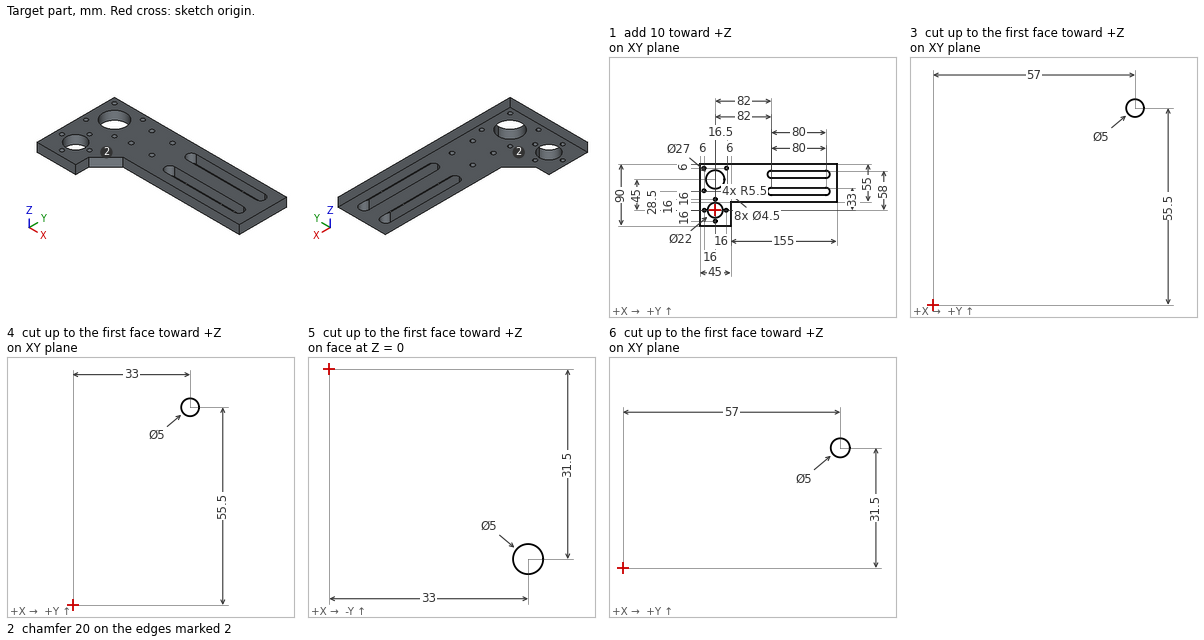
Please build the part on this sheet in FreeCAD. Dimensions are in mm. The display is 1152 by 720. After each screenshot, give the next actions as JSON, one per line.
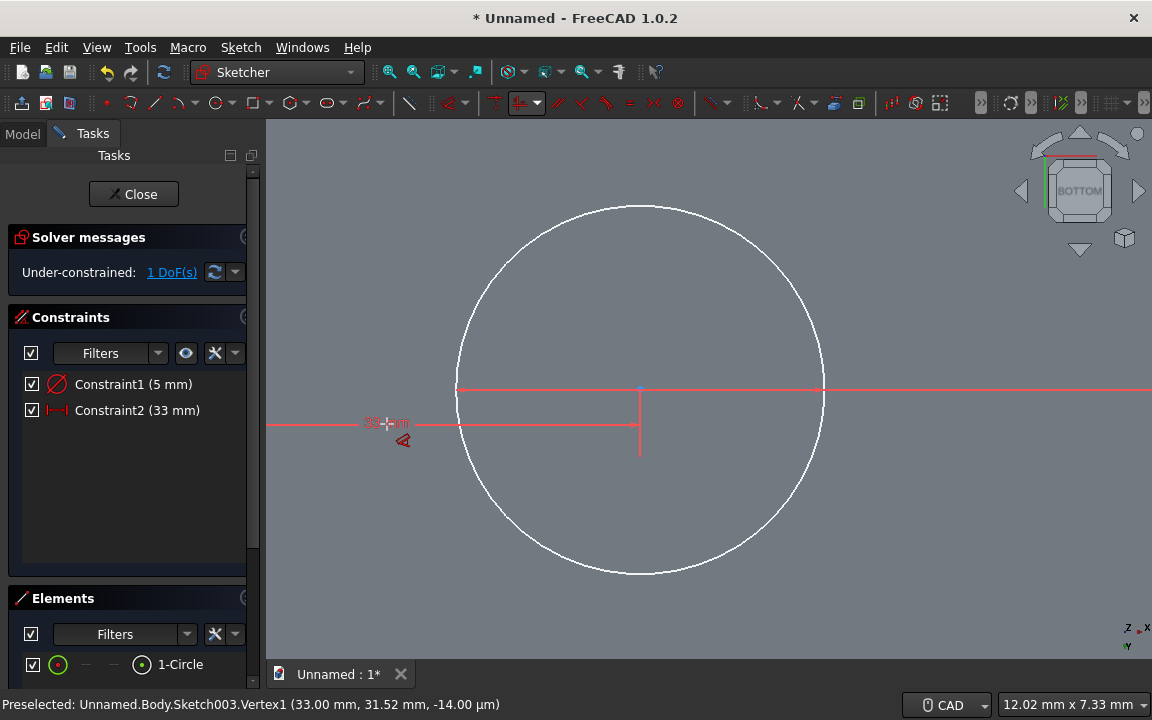
{"action": "left_click", "coordinate": [640, 390]}
{"action": "left_click", "coordinate": [674, 269]}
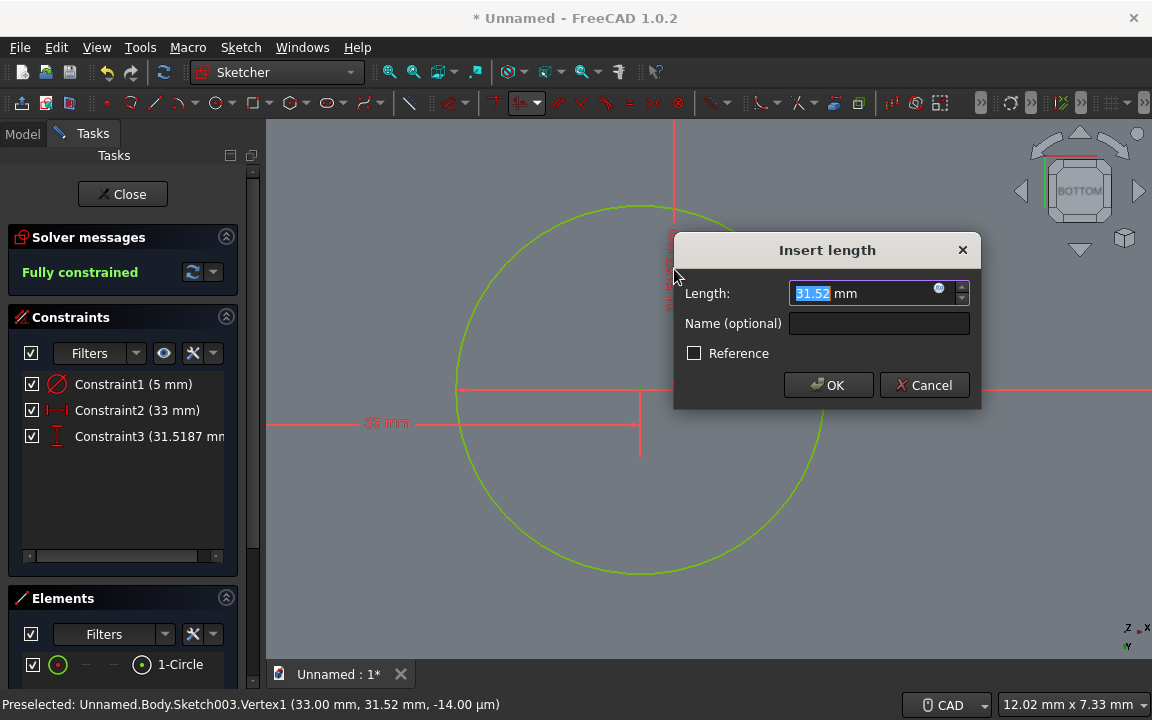
{"action": "type", "text": "31.5"}
{"action": "key", "text": "Return"}
{"action": "key", "text": "Escape"}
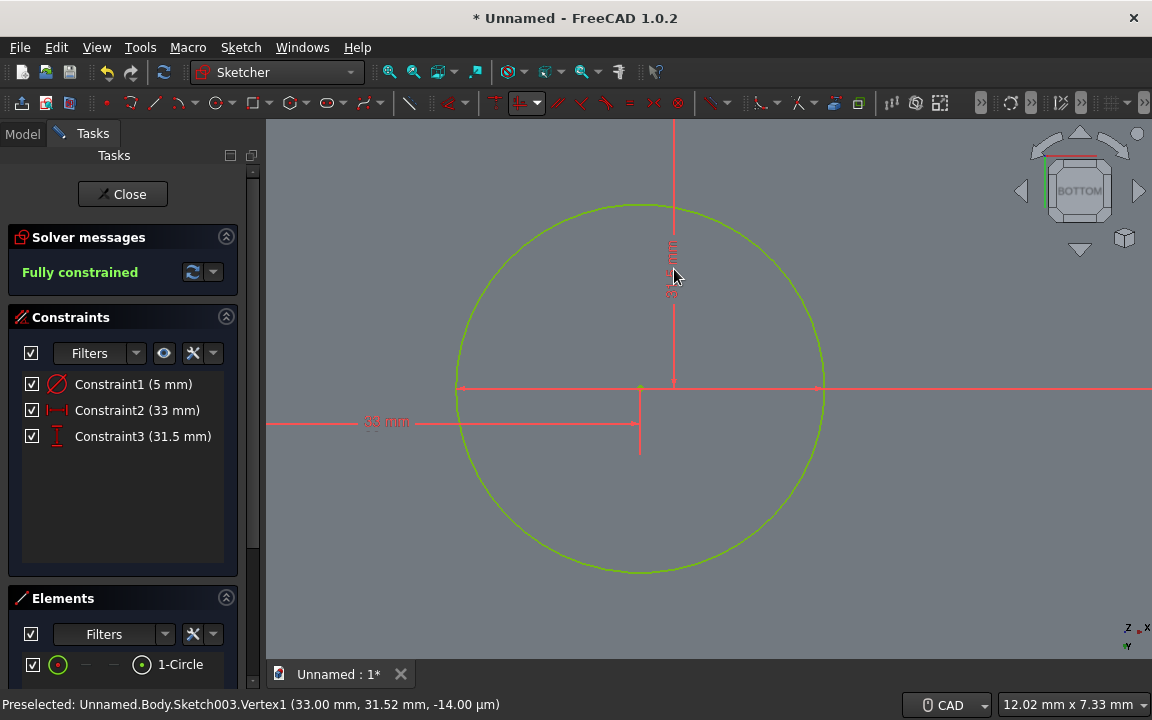
{"action": "left_click", "coordinate": [123, 194]}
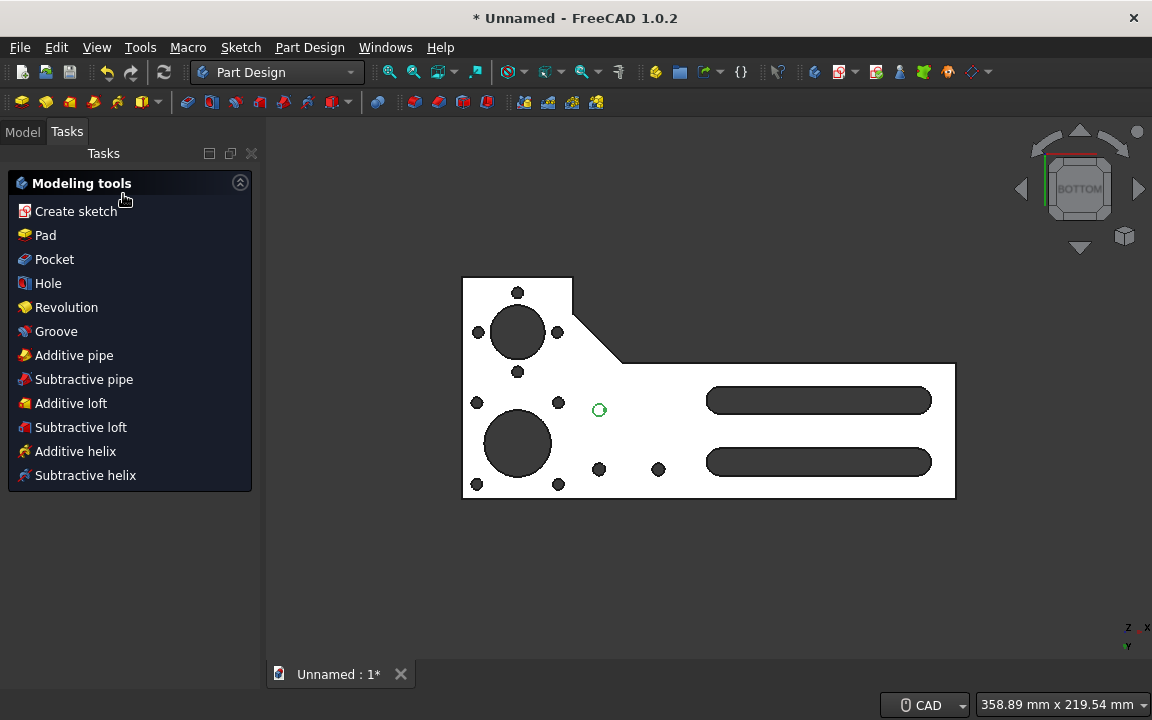
{"action": "left_click", "coordinate": [188, 102]}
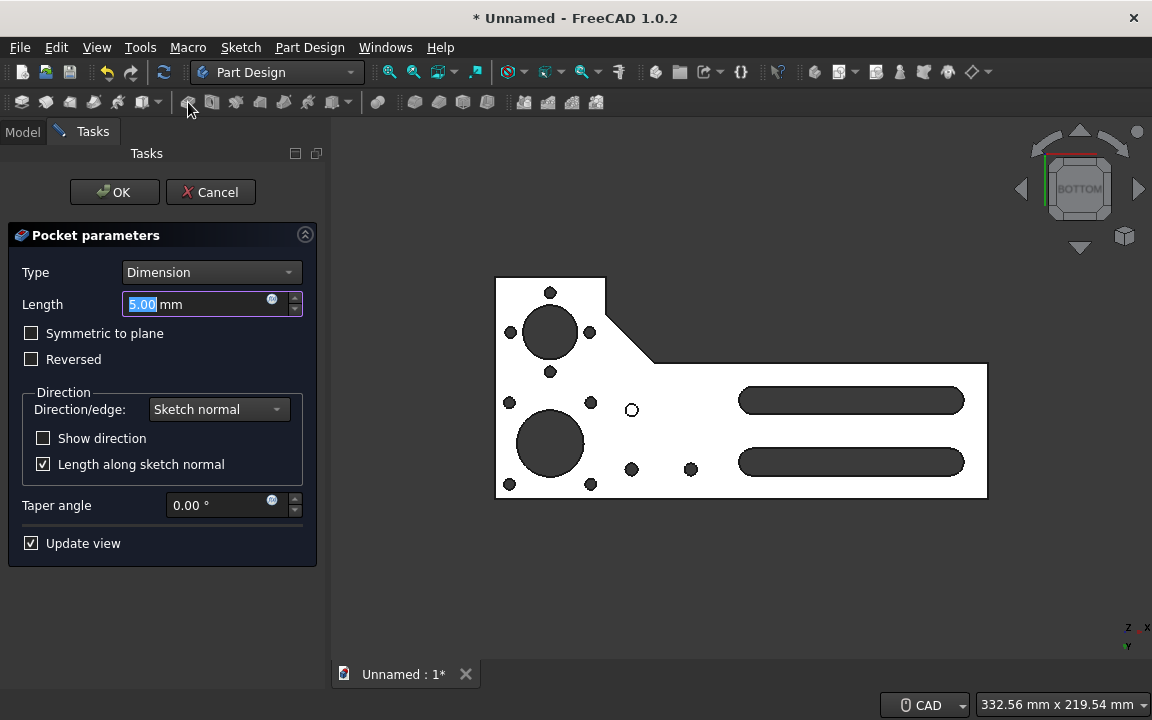
{"action": "left_click", "coordinate": [212, 272]}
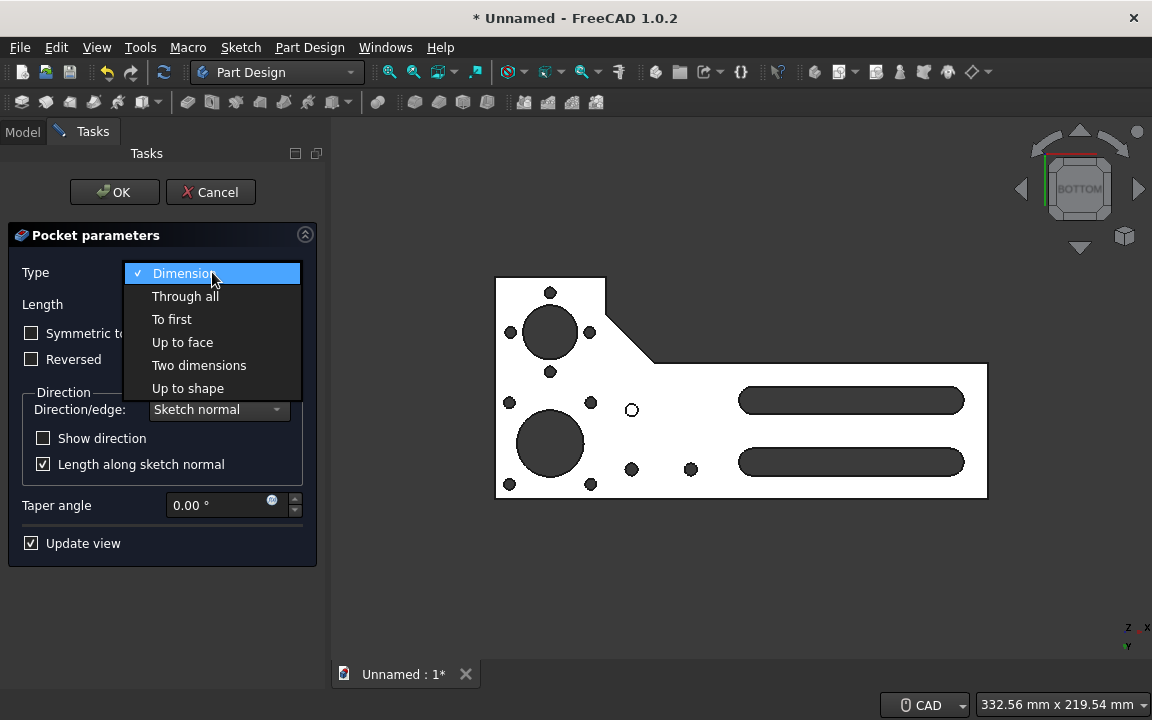
{"action": "left_click", "coordinate": [212, 320]}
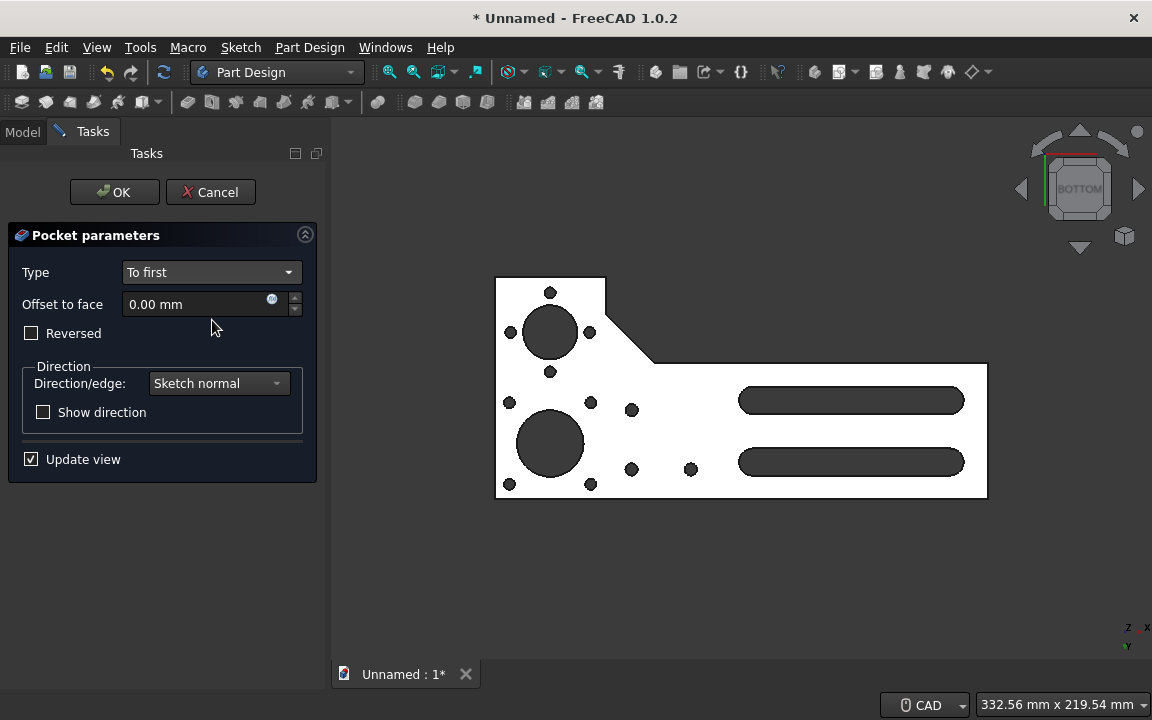
{"action": "left_click", "coordinate": [115, 192]}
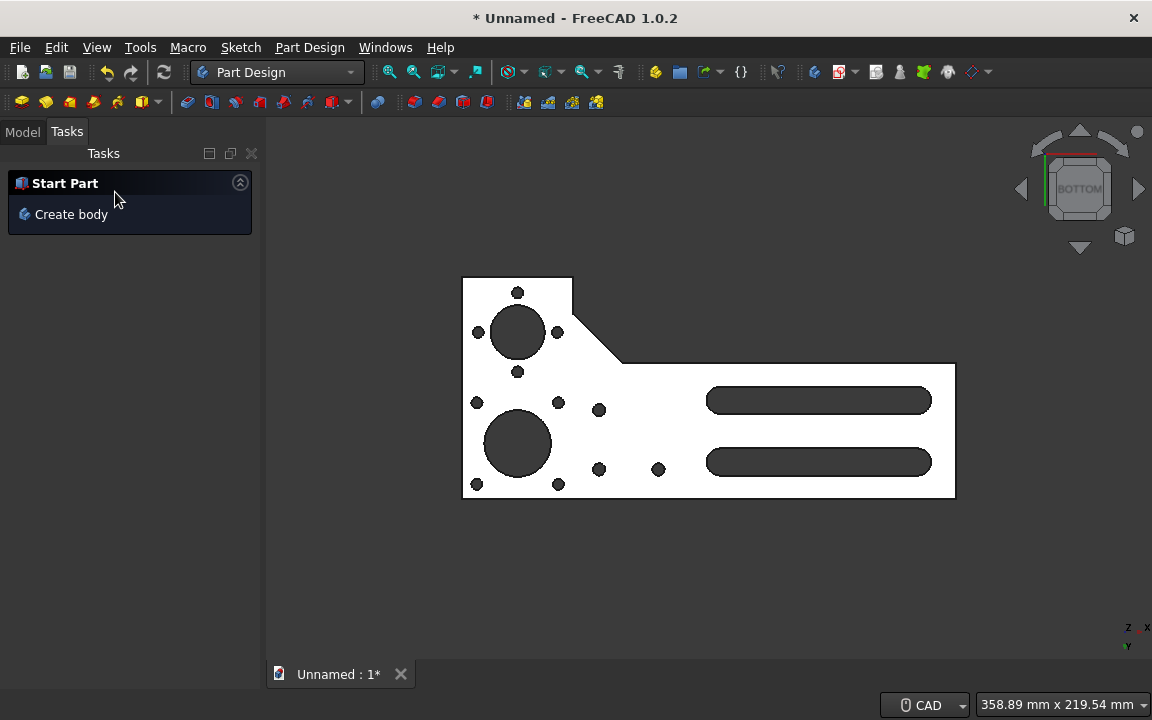
{"action": "left_click", "coordinate": [840, 72]}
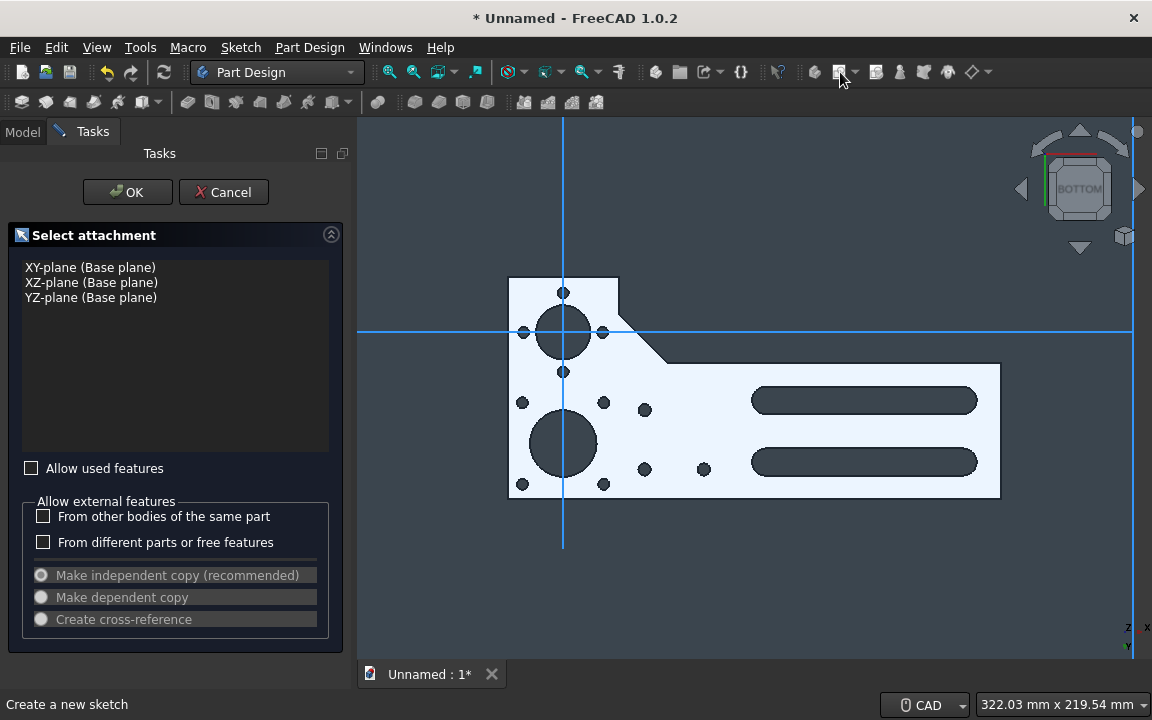
{"action": "left_click", "coordinate": [82, 268]}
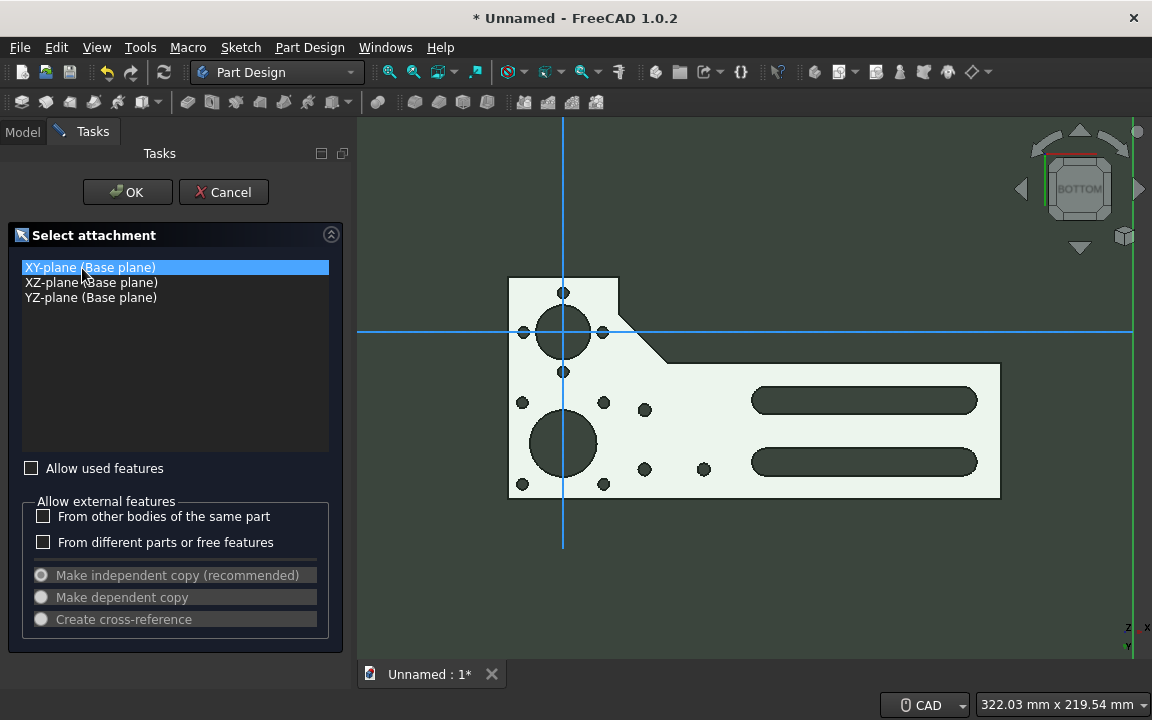
{"action": "left_click", "coordinate": [128, 192]}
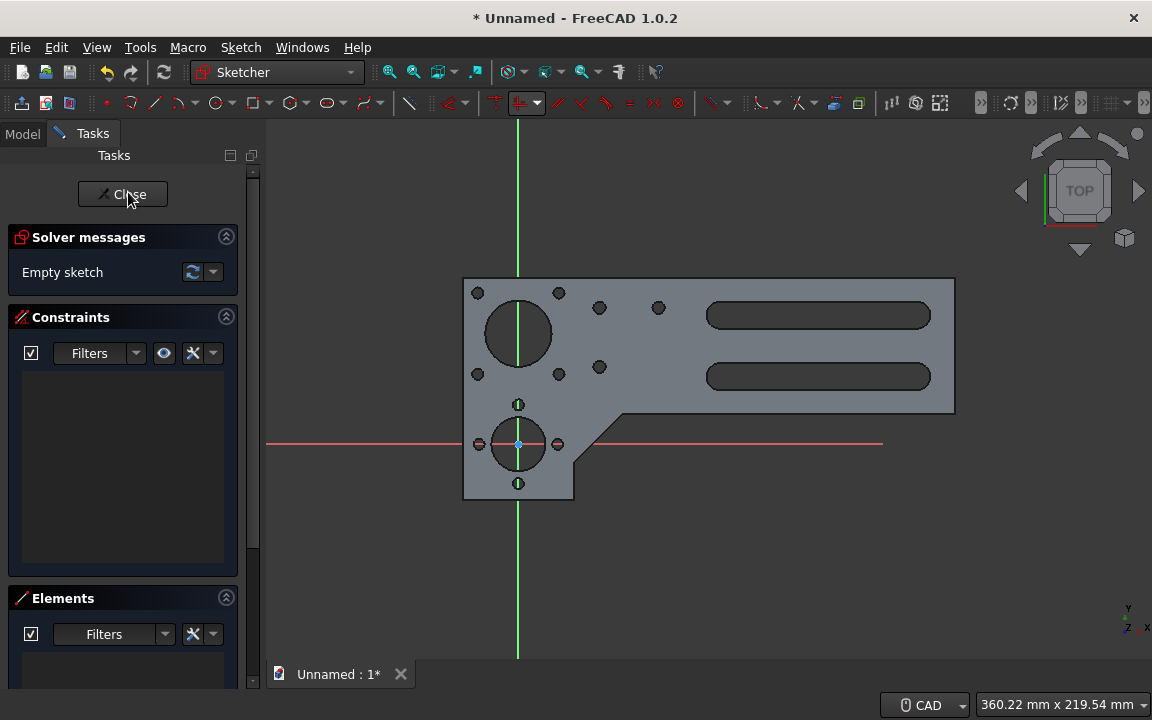
{"action": "key", "text": "q s"}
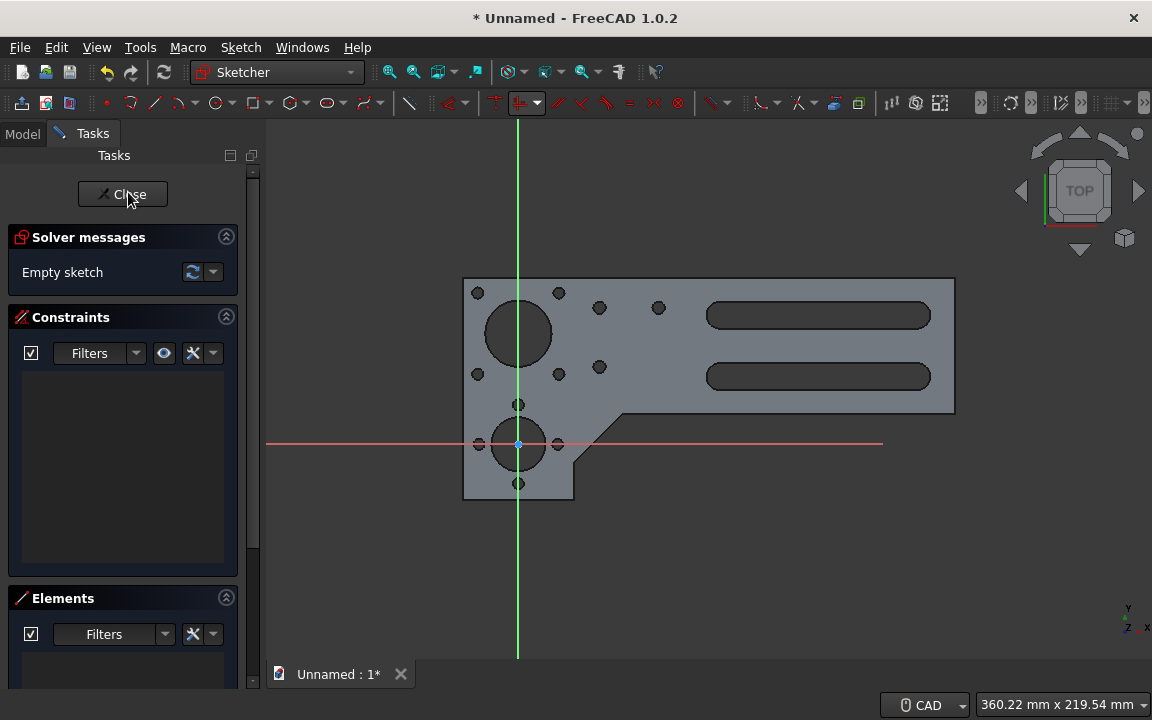
{"action": "scroll", "coordinate": [660, 366], "scroll_direction": "up", "scroll_amount": 15}